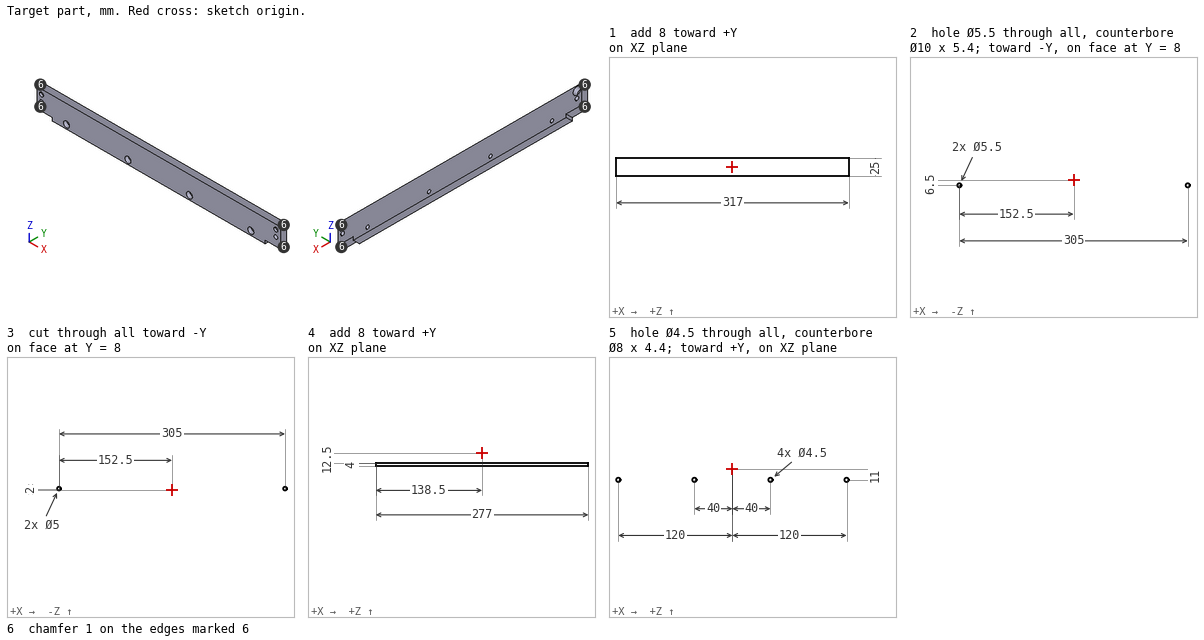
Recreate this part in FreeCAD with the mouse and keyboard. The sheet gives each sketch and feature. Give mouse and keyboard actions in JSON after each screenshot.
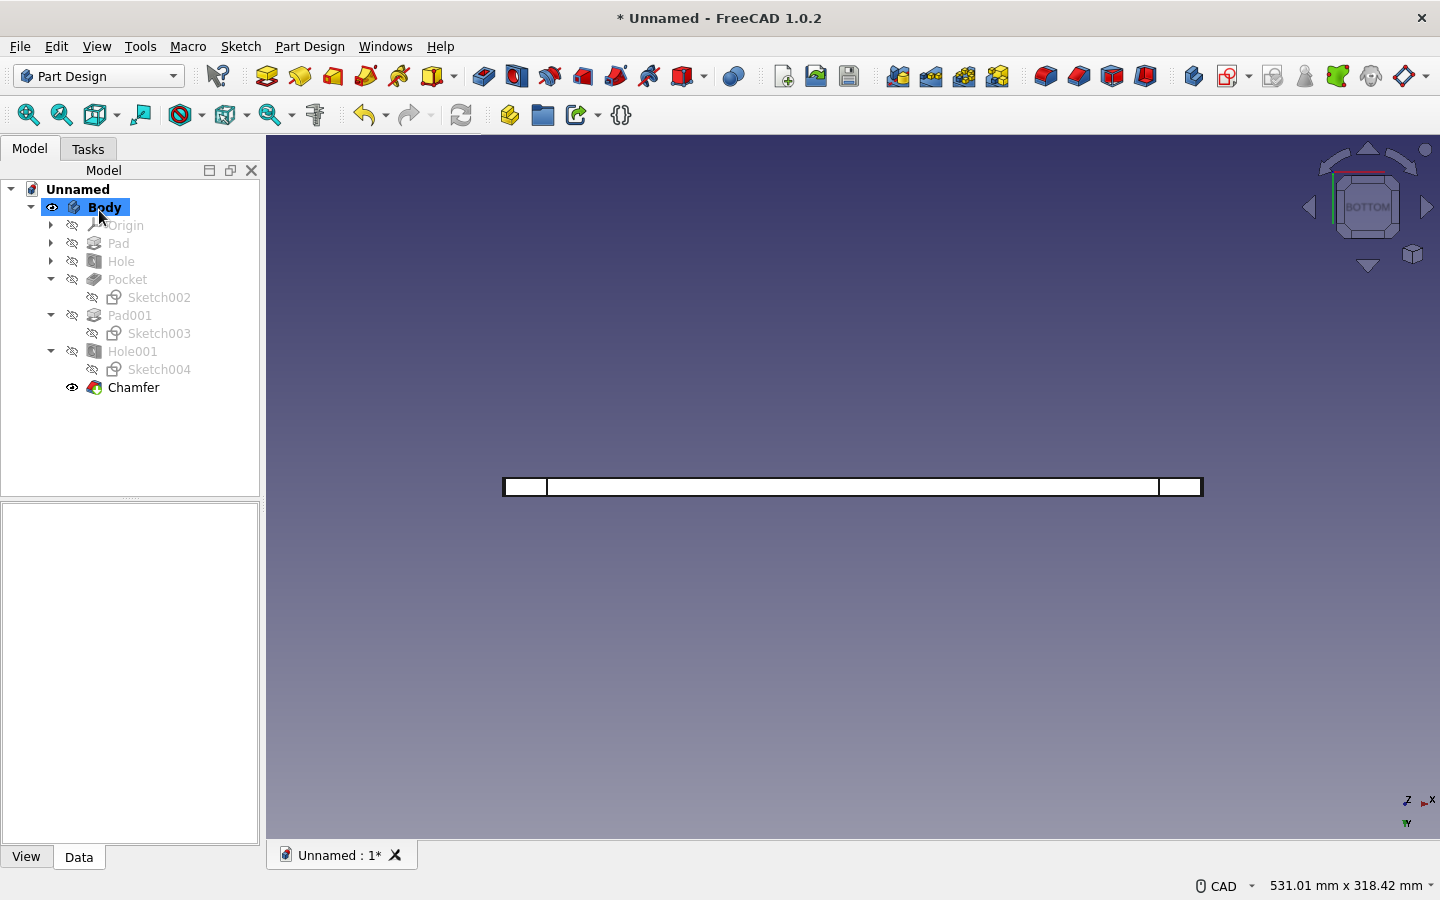
{"action": "key", "text": "0"}